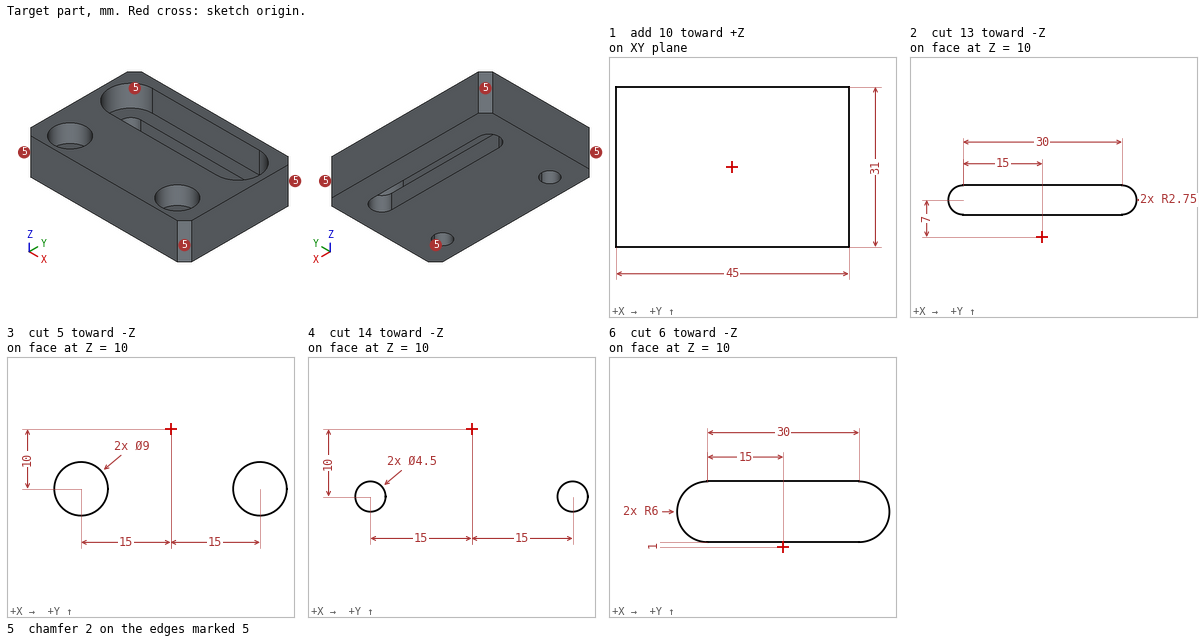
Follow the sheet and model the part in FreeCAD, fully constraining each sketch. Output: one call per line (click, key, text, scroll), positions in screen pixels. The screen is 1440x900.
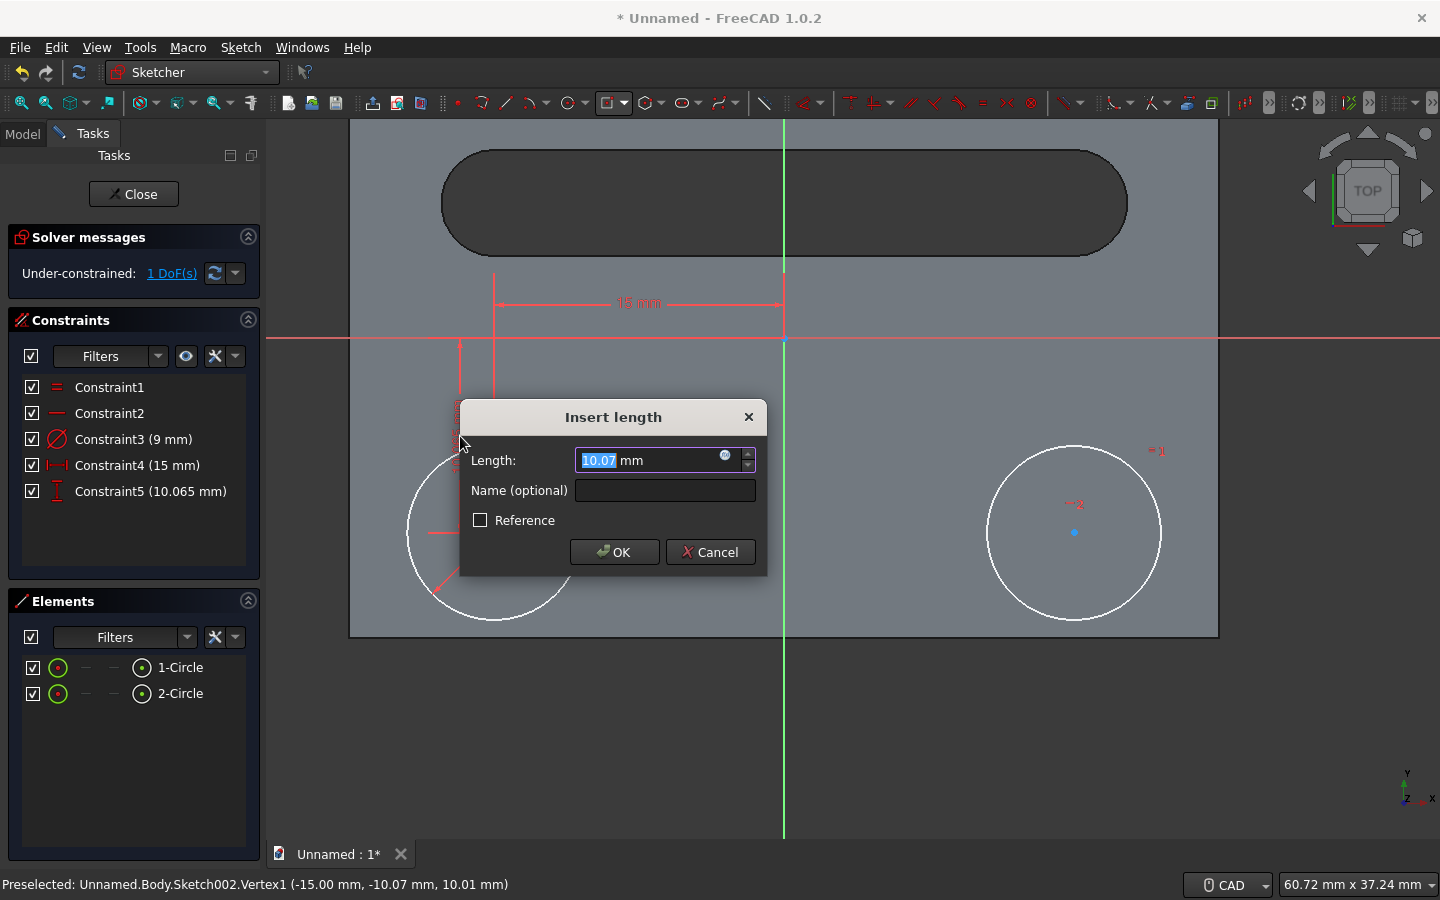
text(10)
key(Return)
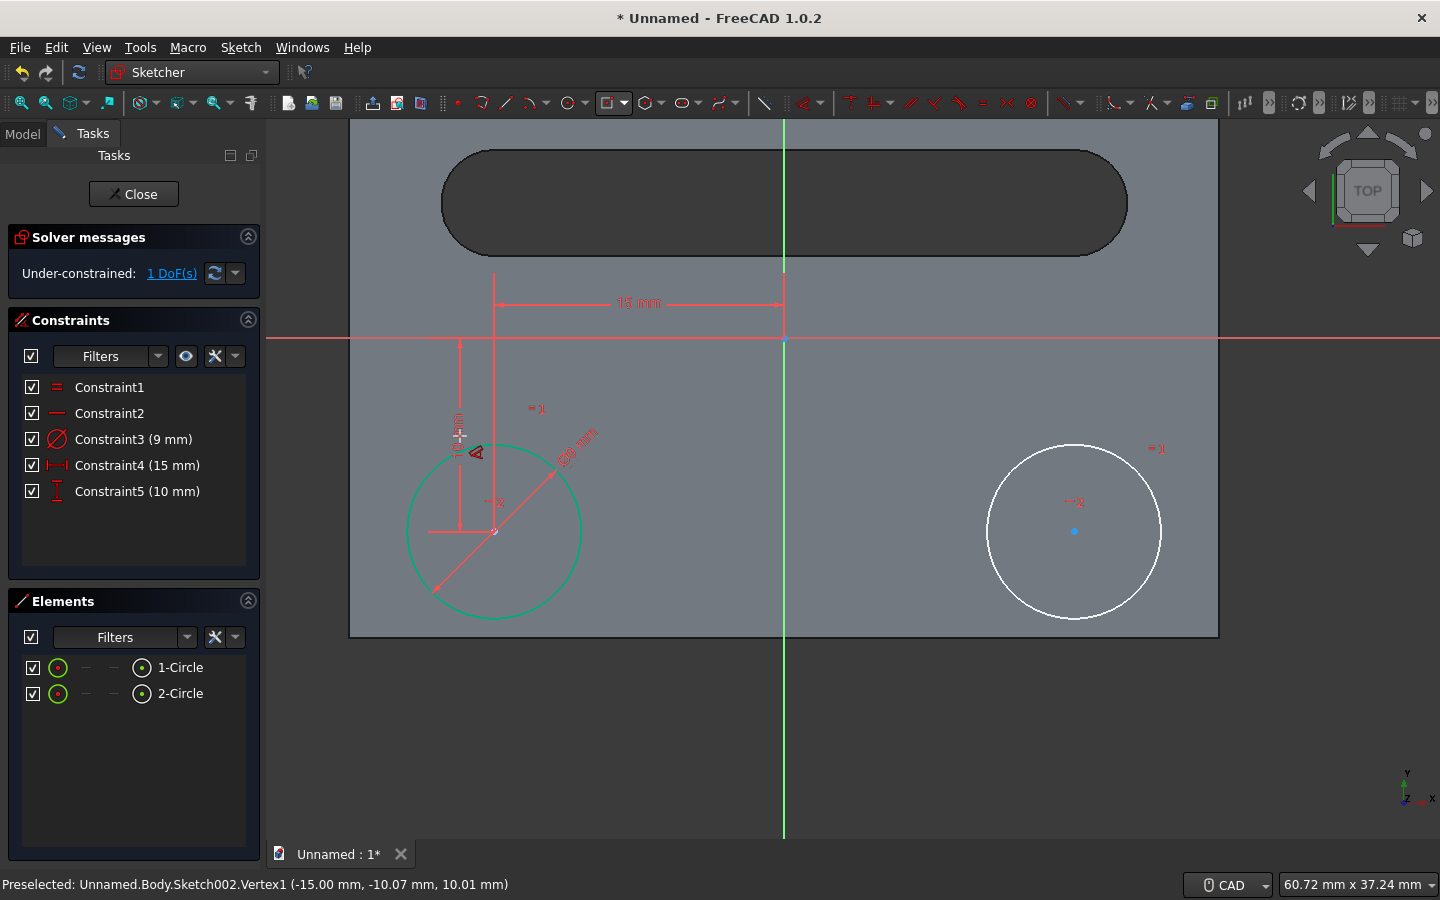
click(1074, 532)
click(929, 304)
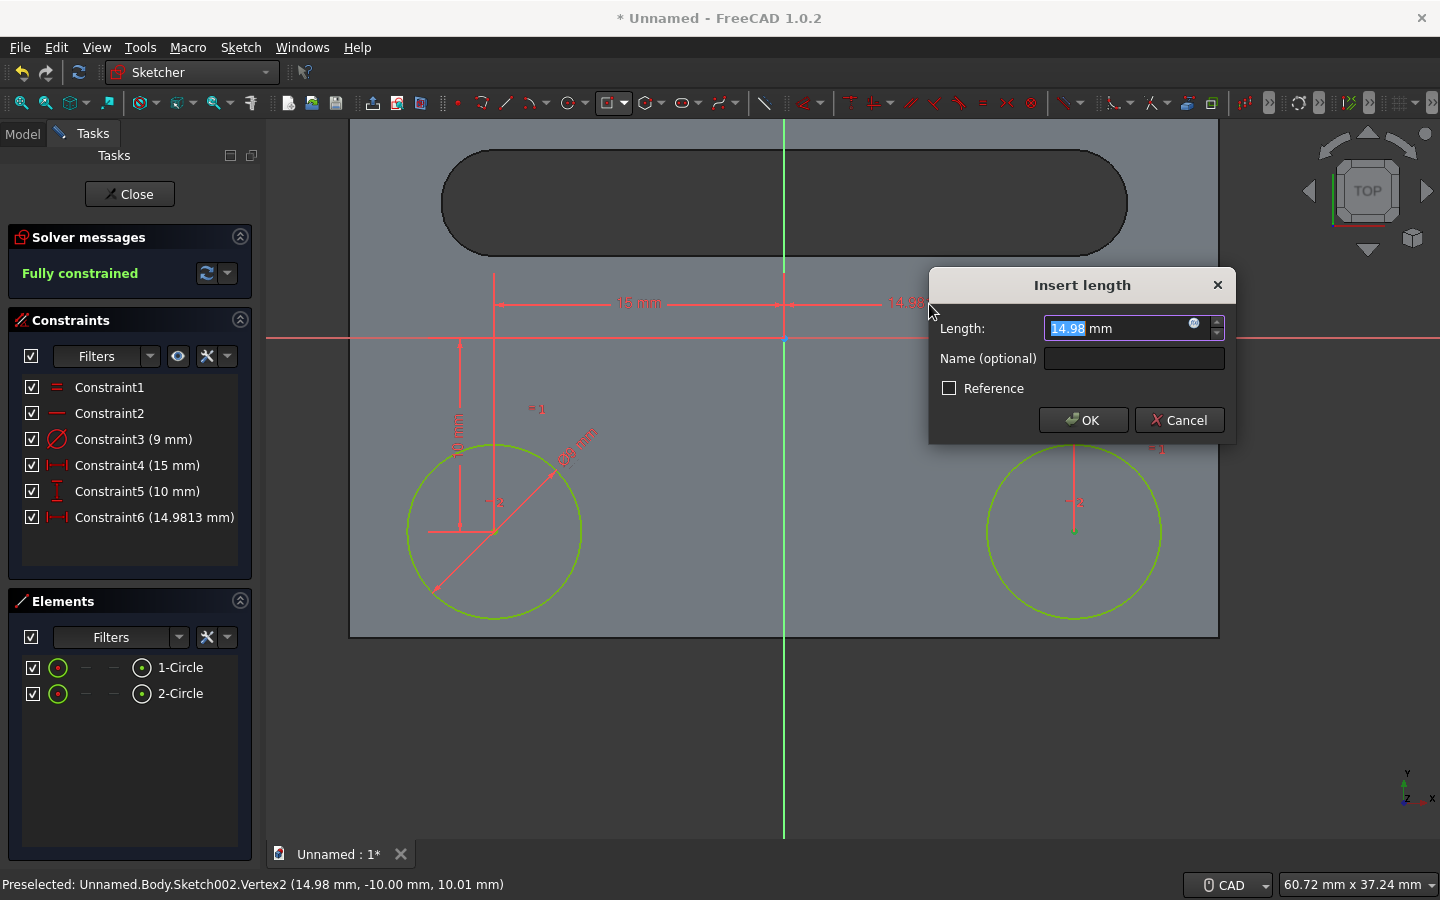
text(15)
key(Return)
key(Escape)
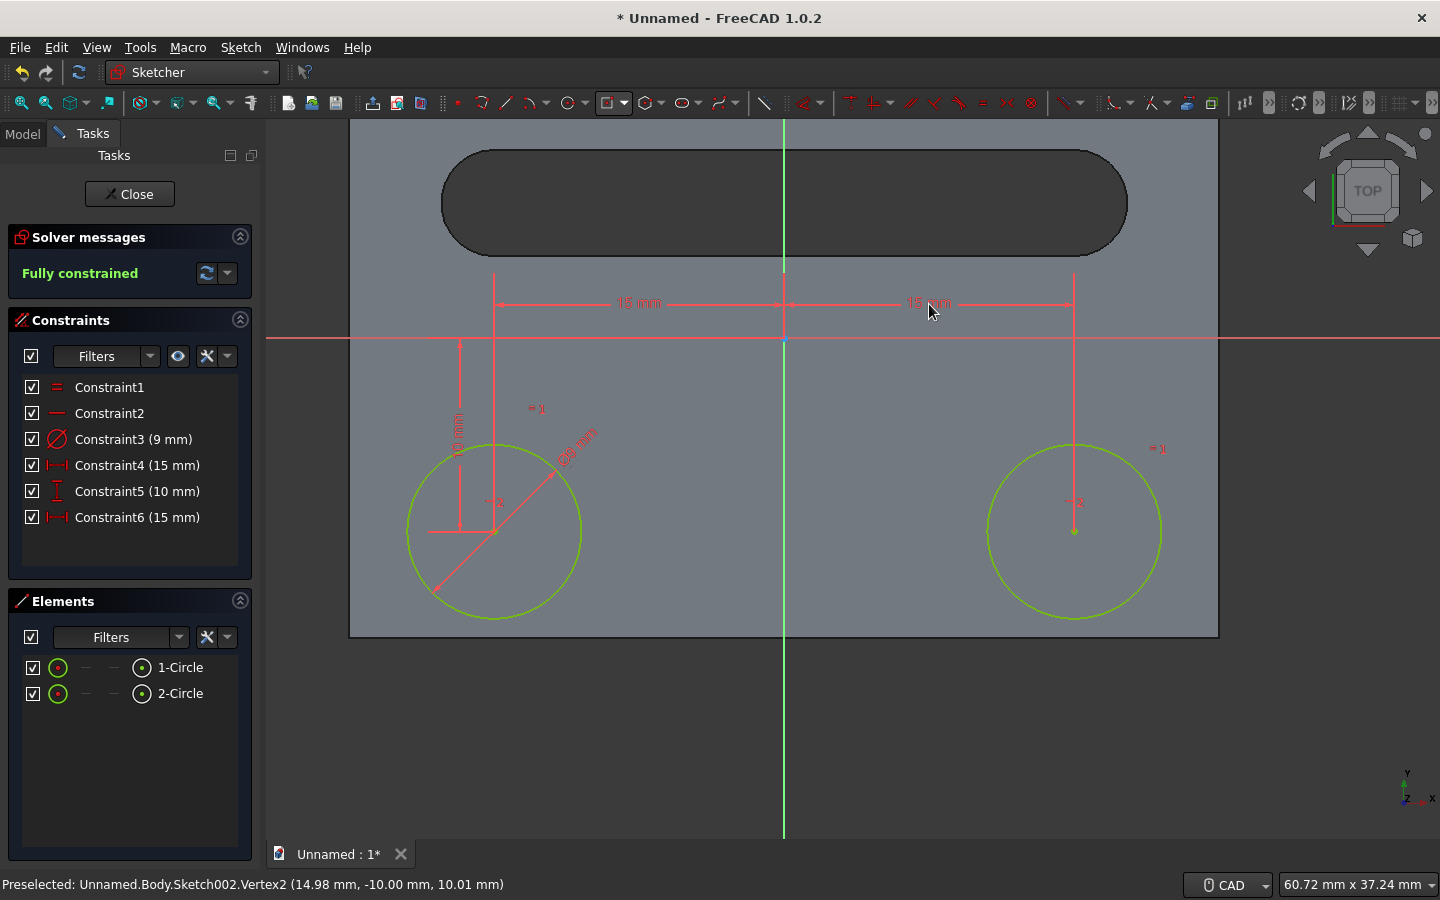
click(130, 194)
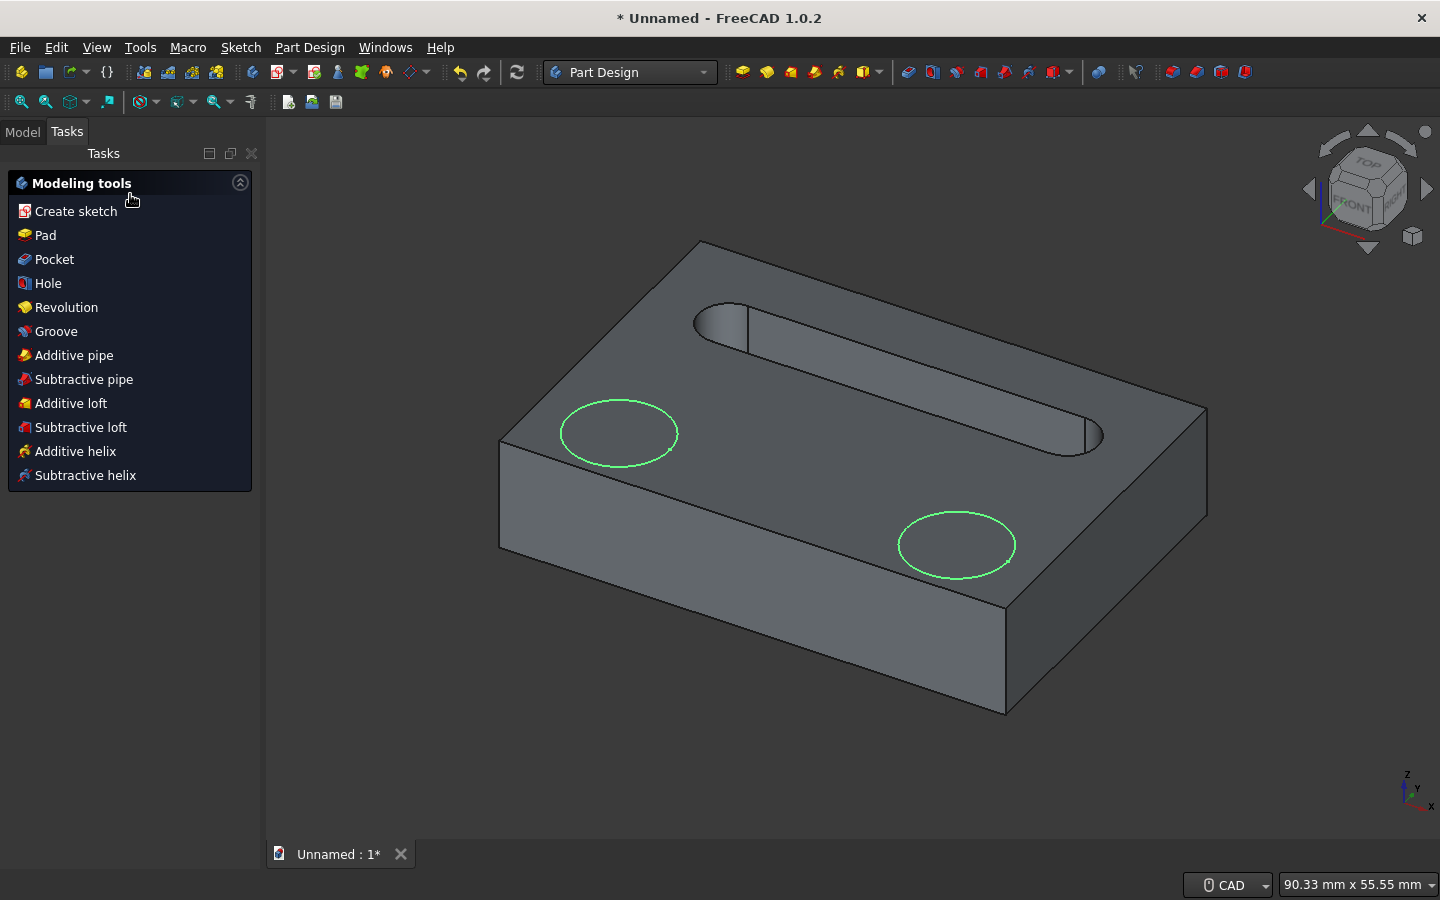
click(910, 72)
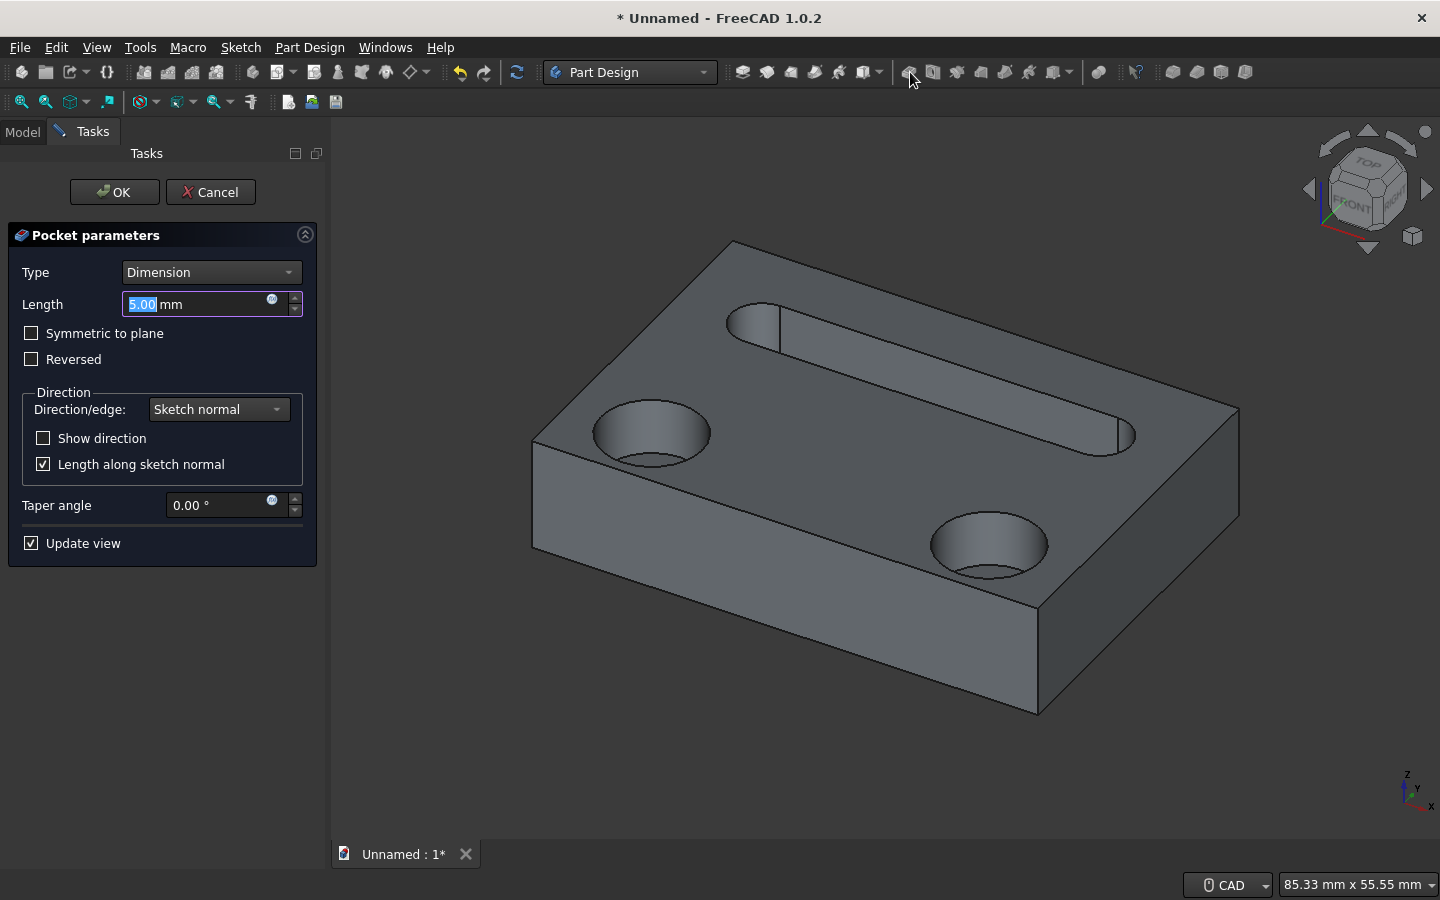
text(5)
key(Tab)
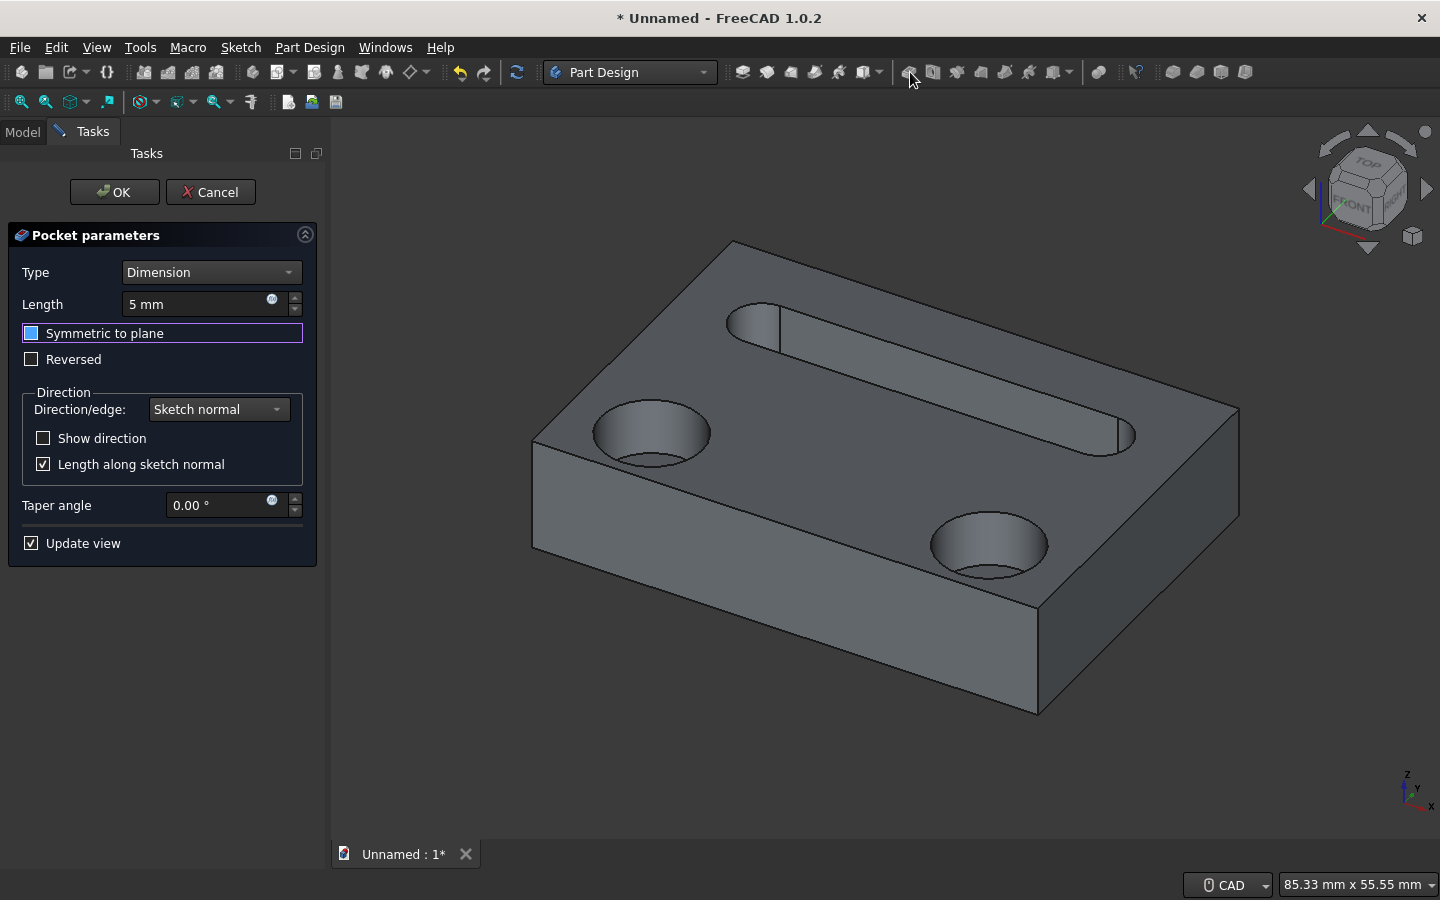
click(115, 192)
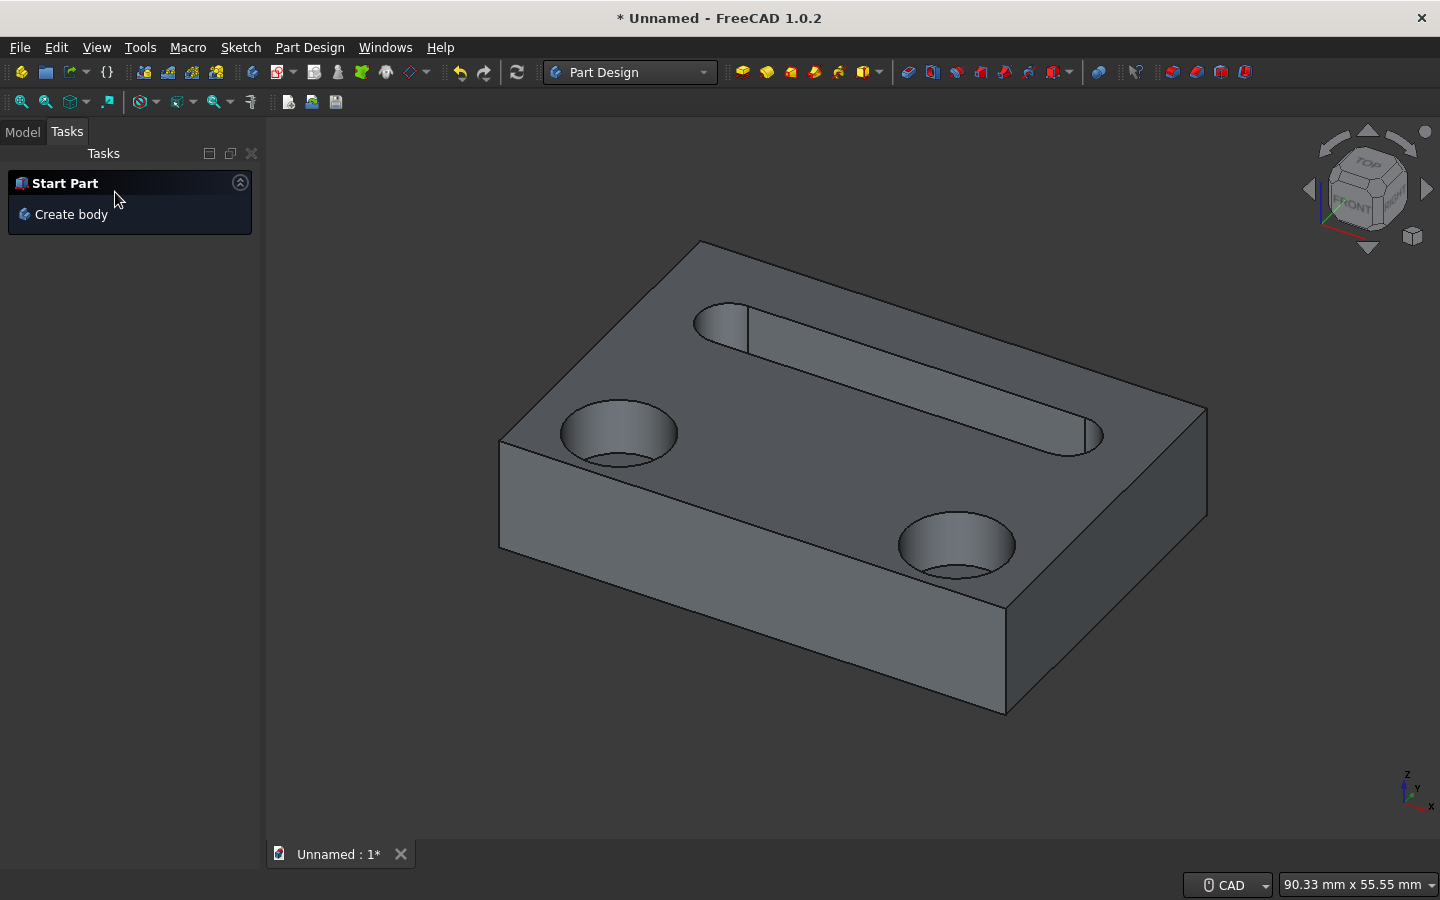
click(824, 452)